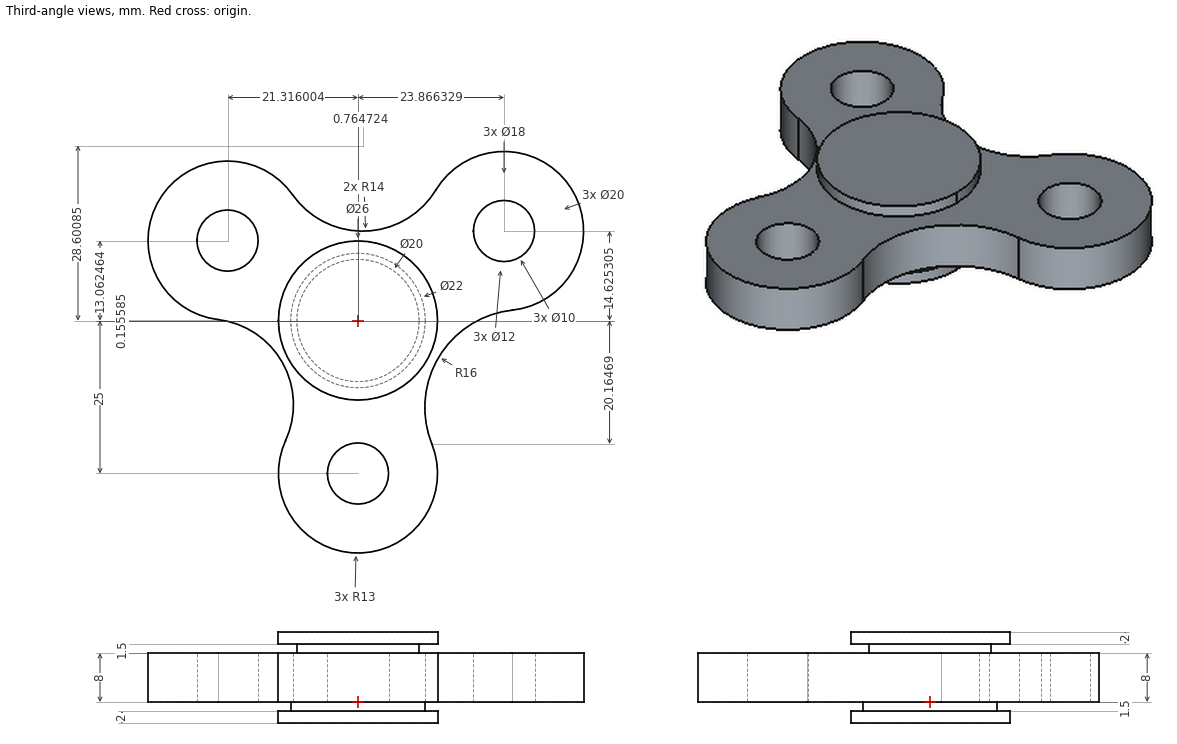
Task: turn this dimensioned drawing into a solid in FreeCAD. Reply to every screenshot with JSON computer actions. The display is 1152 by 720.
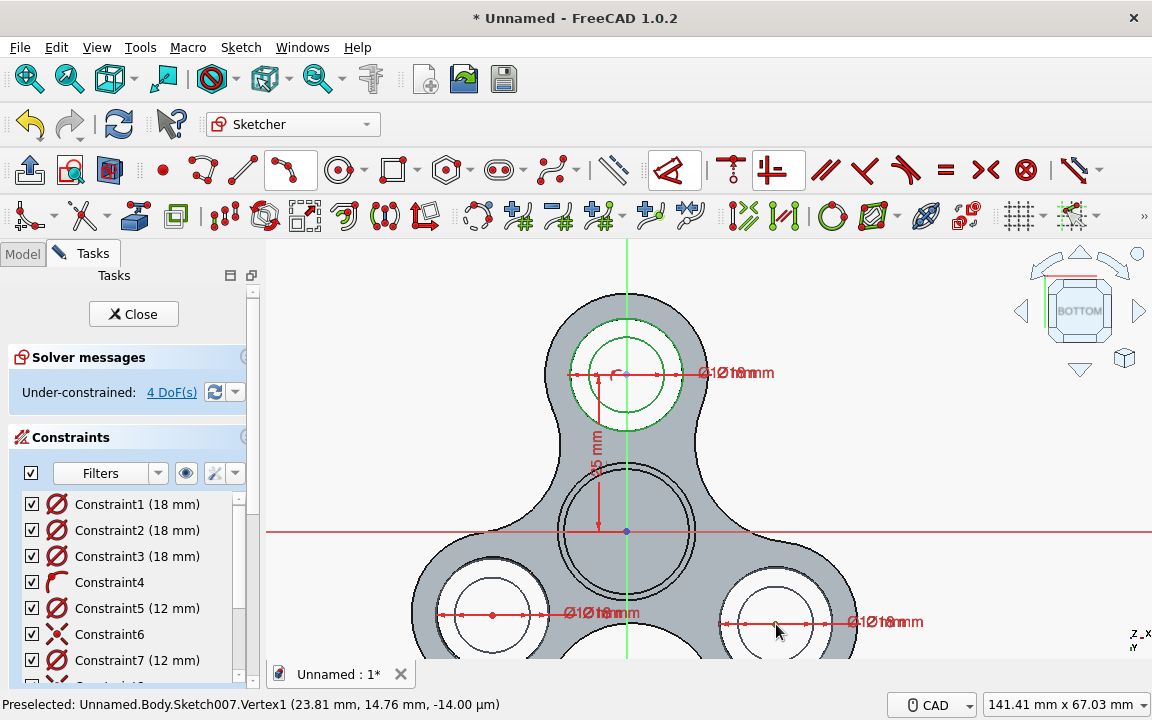
{"action": "left_click", "coordinate": [696, 170]}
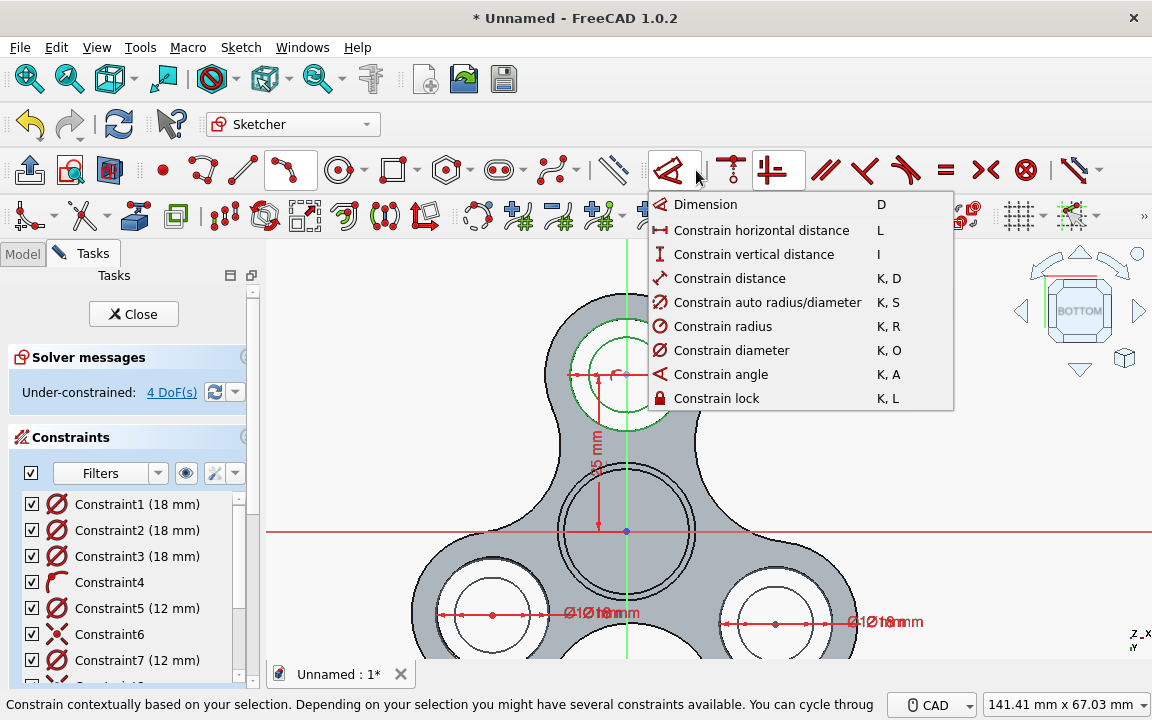
{"action": "left_click", "coordinate": [801, 230]}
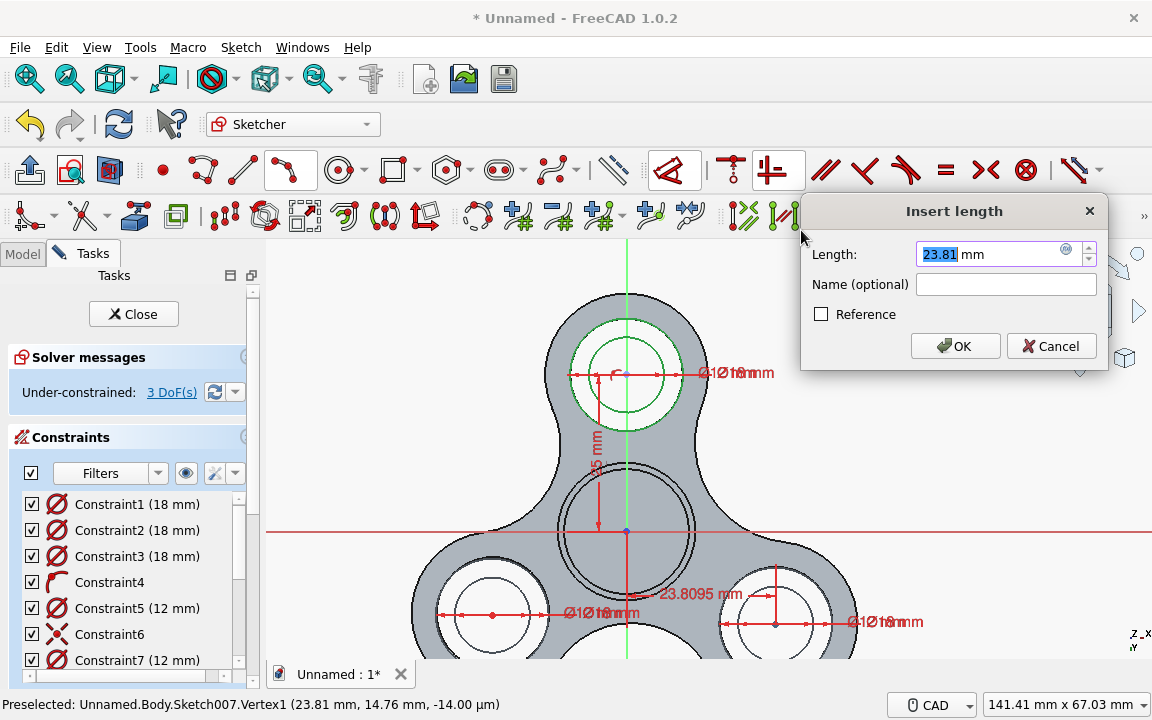
{"action": "type", "text": "23.866329"}
{"action": "key", "text": "Return"}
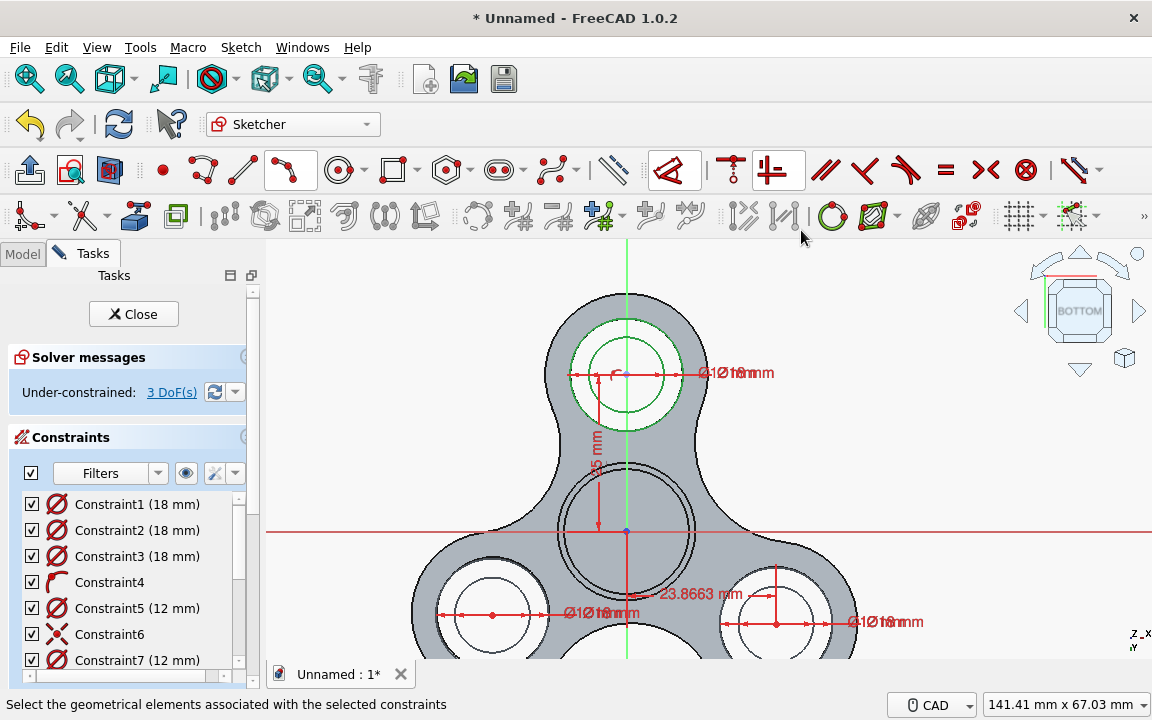
{"action": "left_click", "coordinate": [776, 624]}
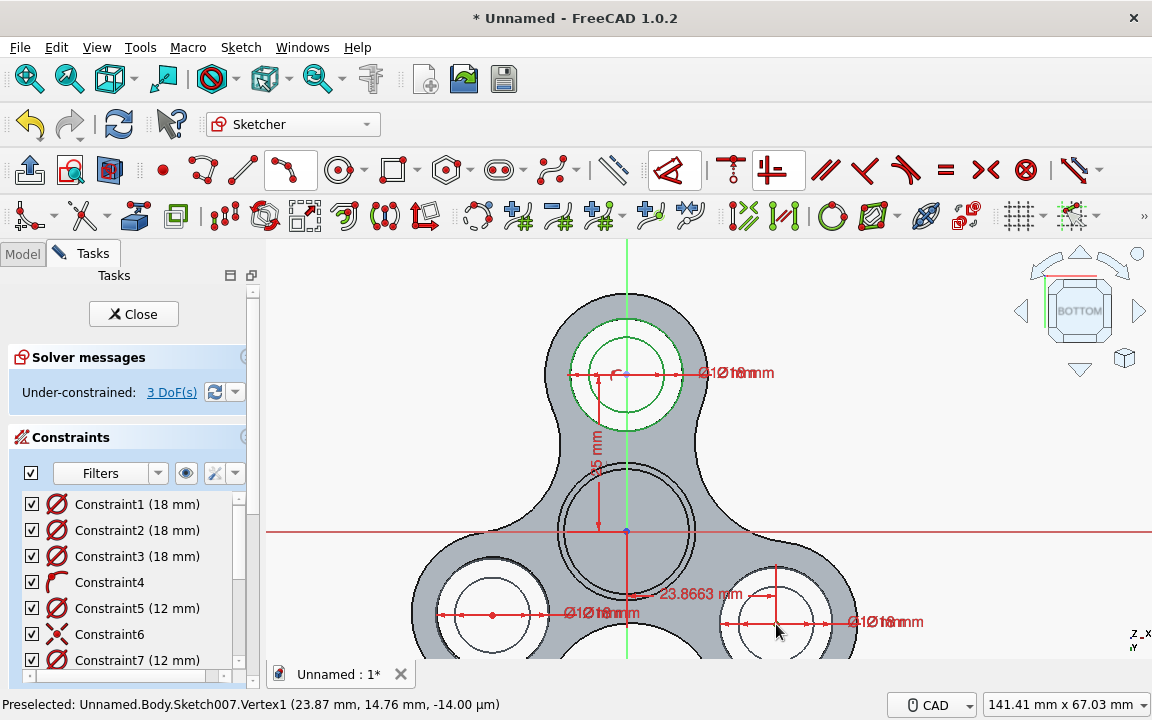
{"action": "left_click", "coordinate": [696, 170]}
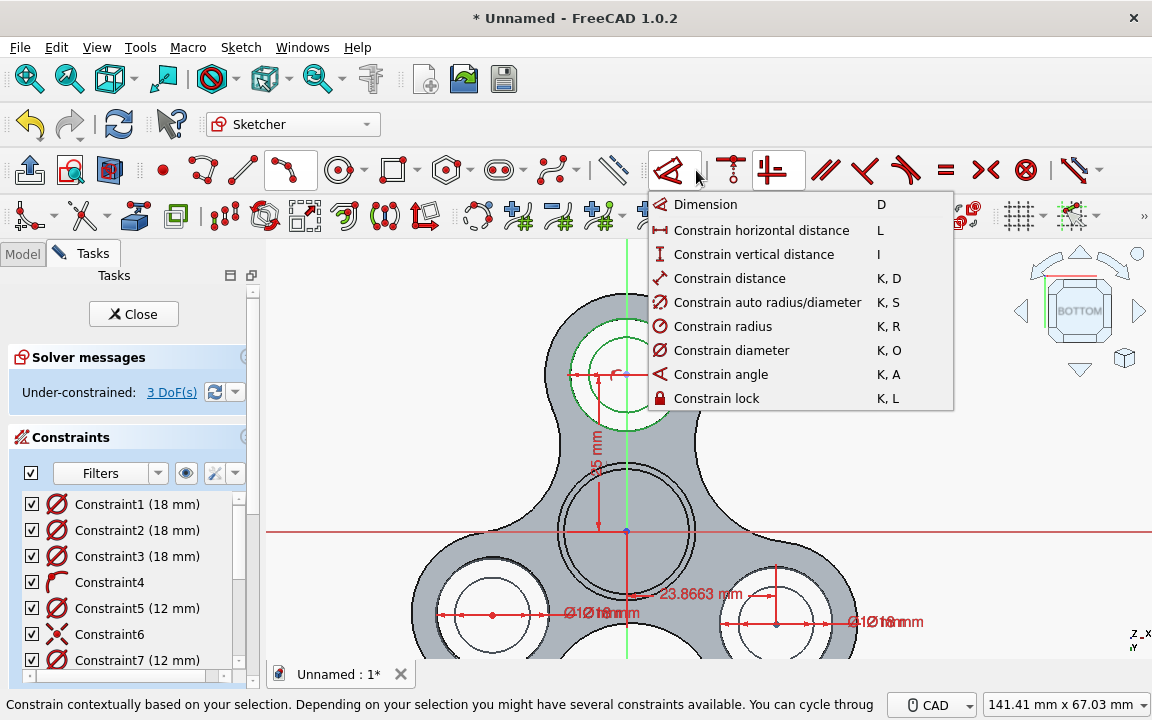
{"action": "left_click", "coordinate": [801, 254]}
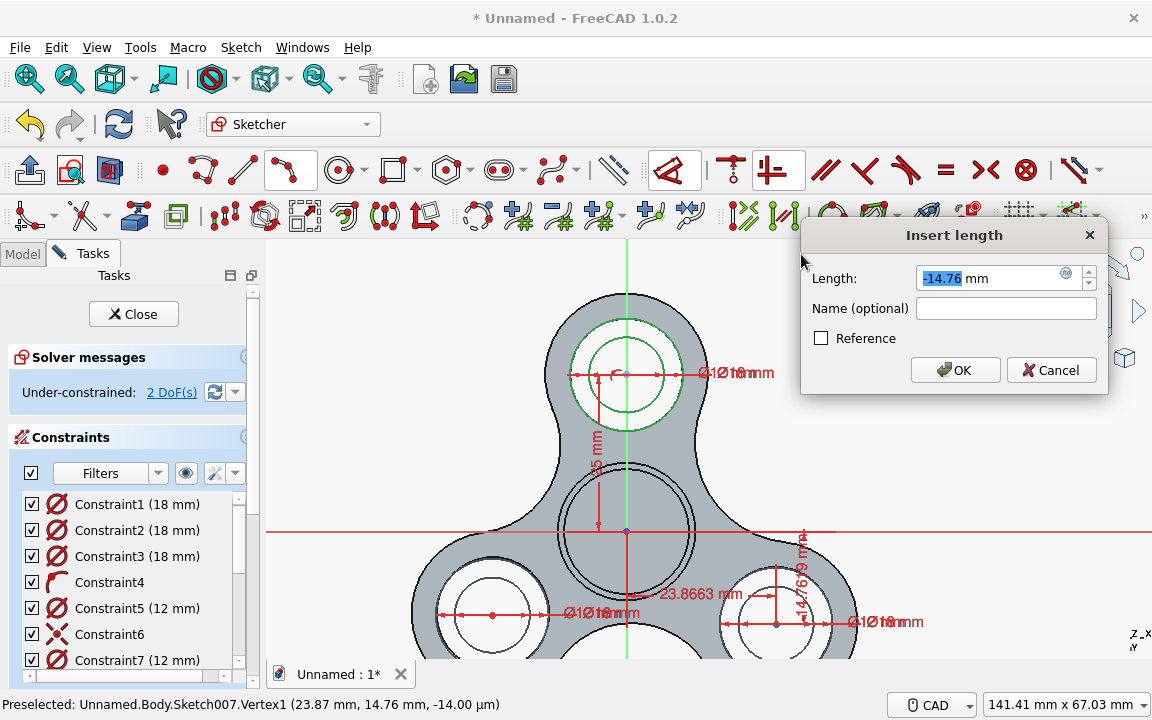
{"action": "type", "text": "-14.625305"}
{"action": "key", "text": "Return"}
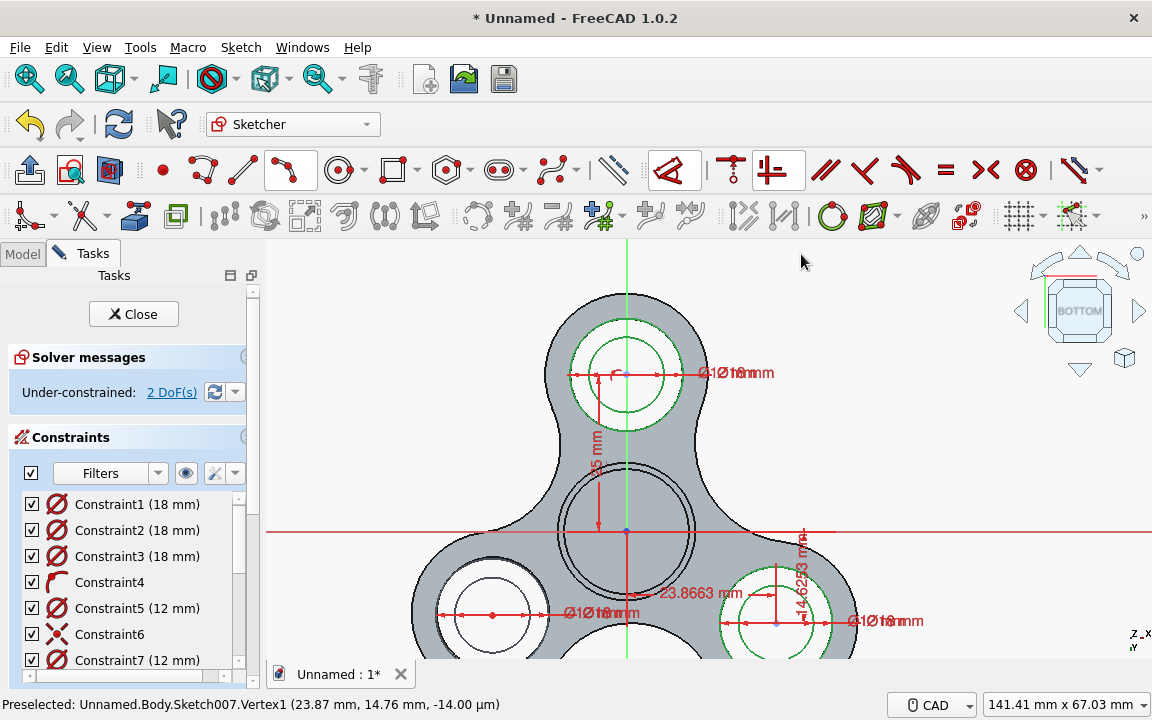
{"action": "left_click", "coordinate": [492, 615]}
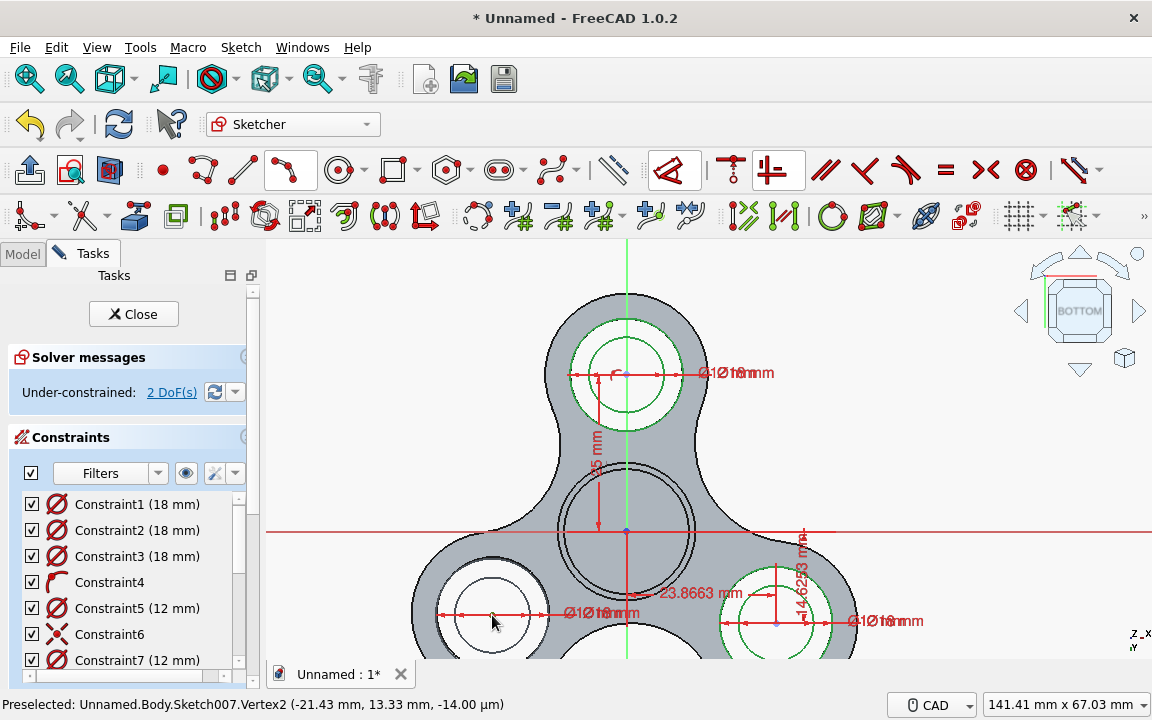
{"action": "left_click", "coordinate": [696, 170]}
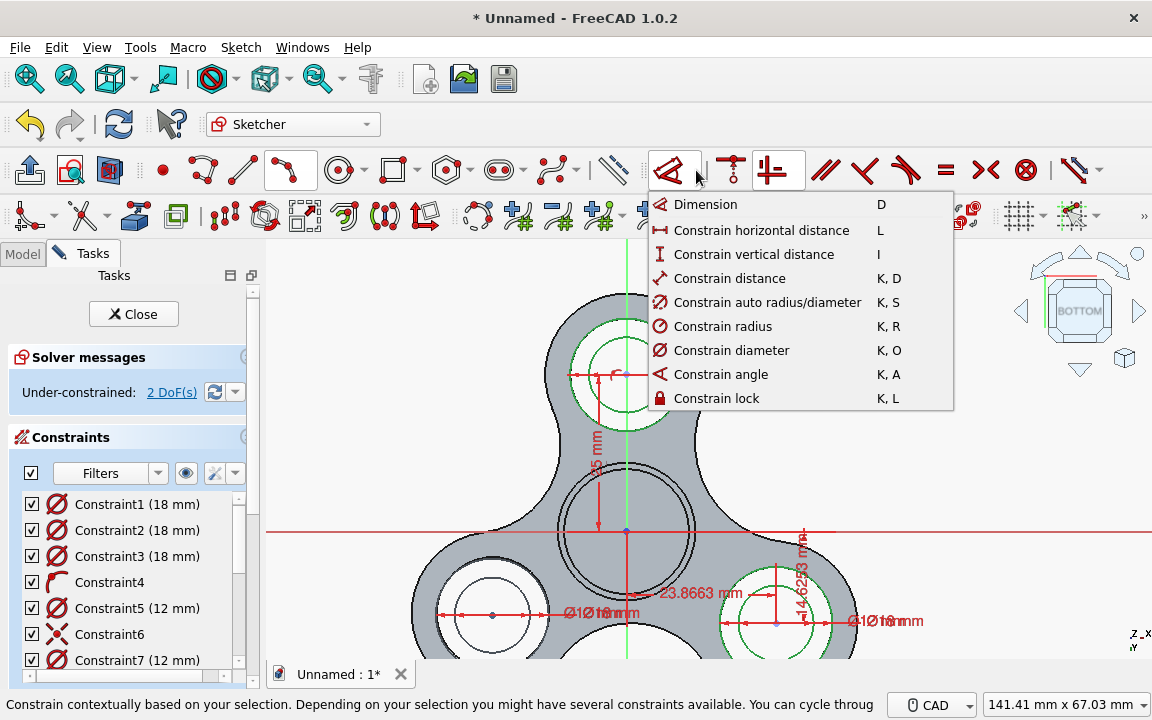
{"action": "left_click", "coordinate": [801, 230]}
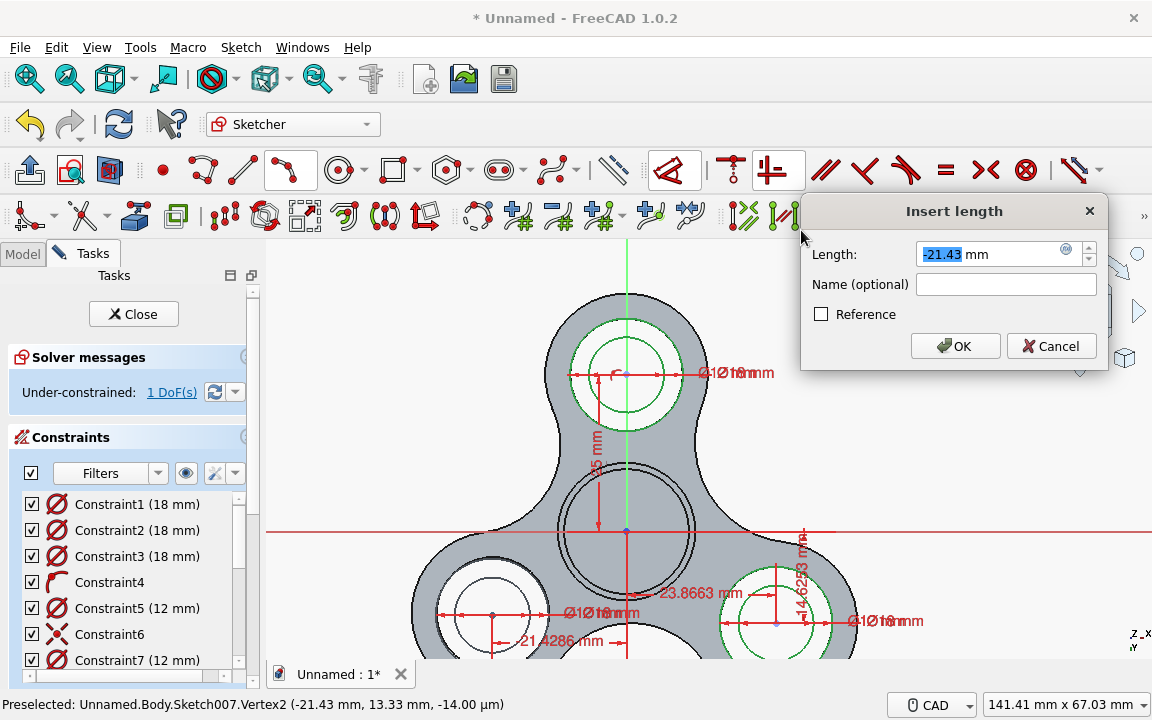
{"action": "type", "text": "-21.316004"}
{"action": "key", "text": "Return"}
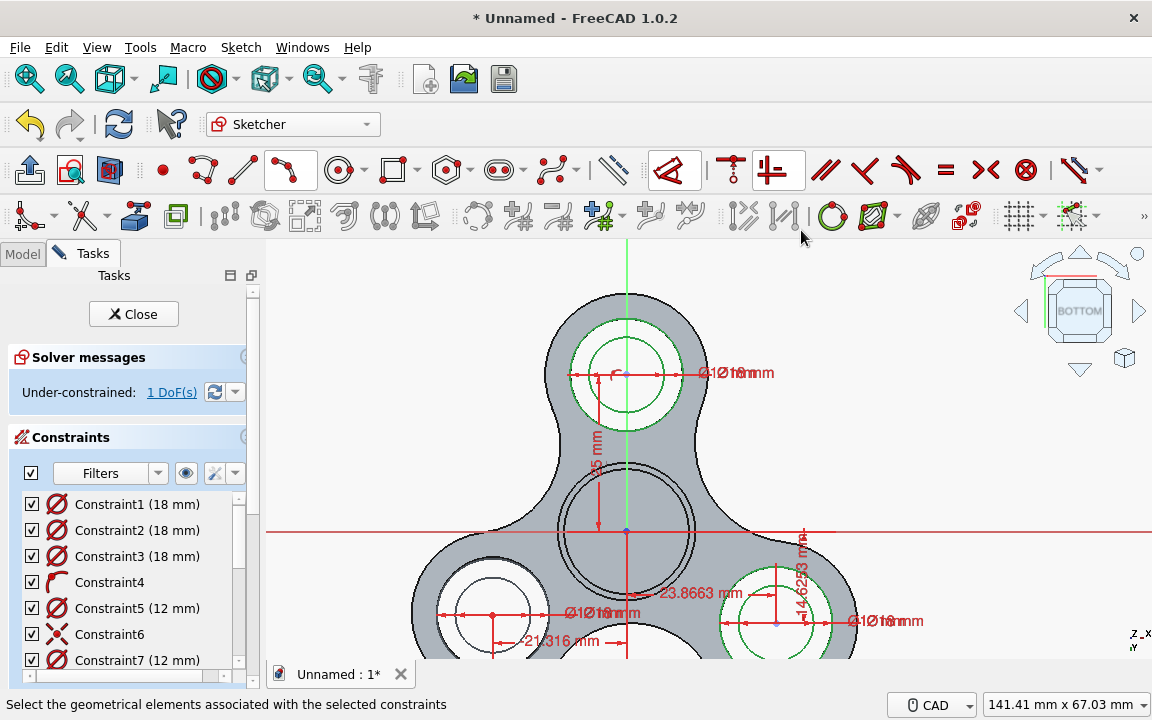
{"action": "left_click", "coordinate": [493, 615]}